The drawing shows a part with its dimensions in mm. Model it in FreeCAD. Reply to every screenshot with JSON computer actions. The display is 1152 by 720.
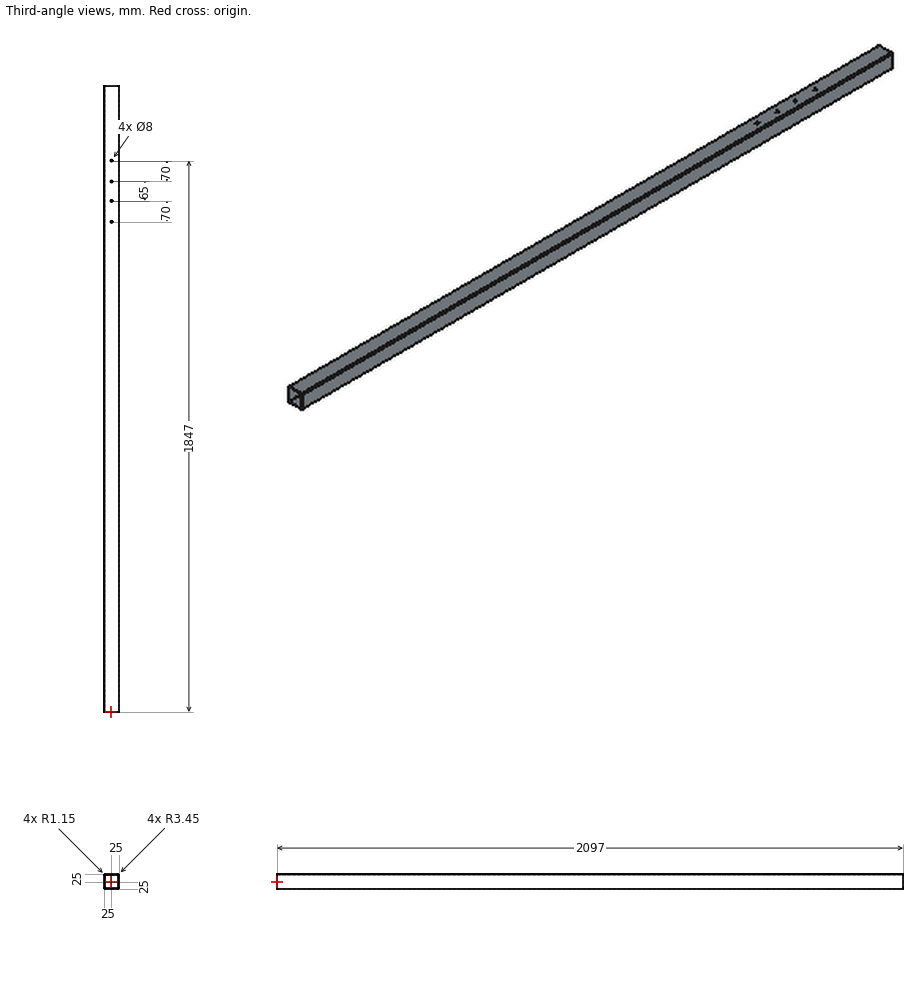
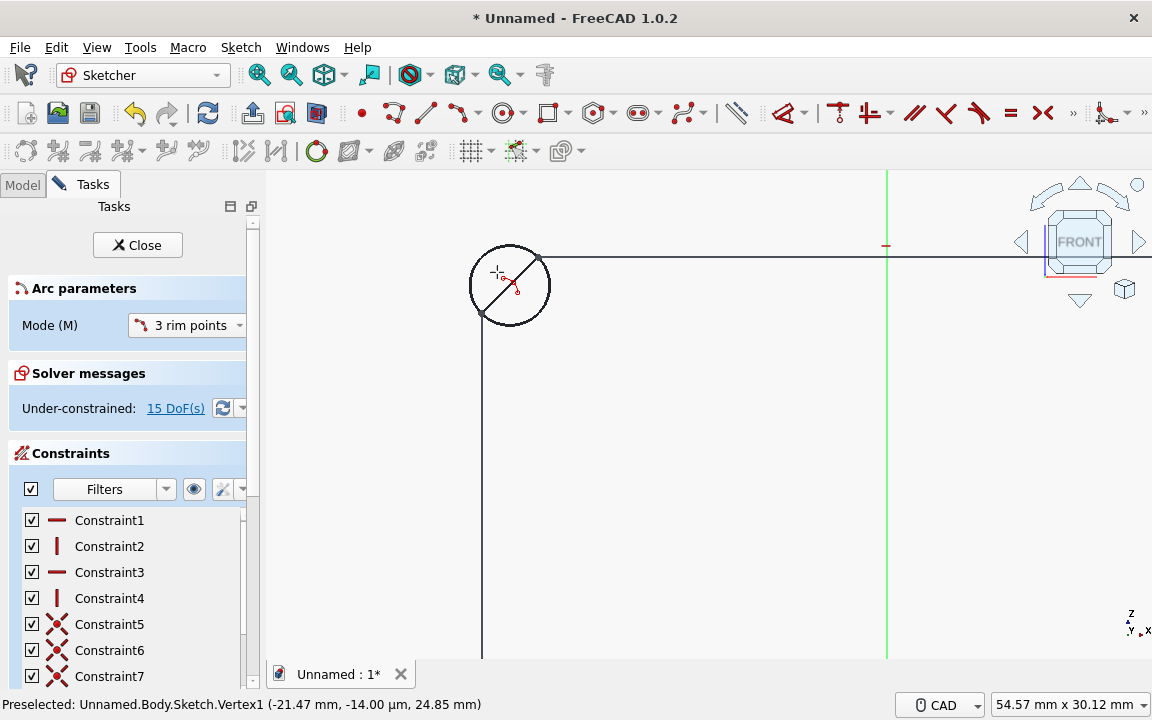
{"action": "left_click", "coordinate": [497, 271]}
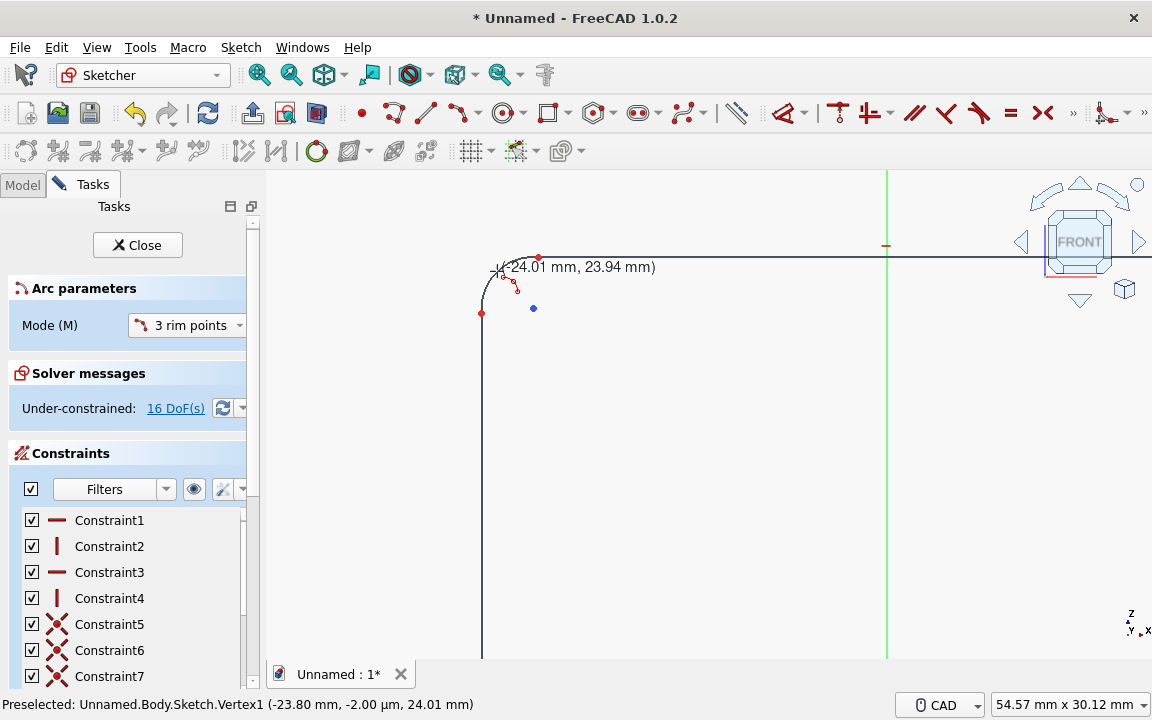
{"action": "left_click", "coordinate": [426, 114]}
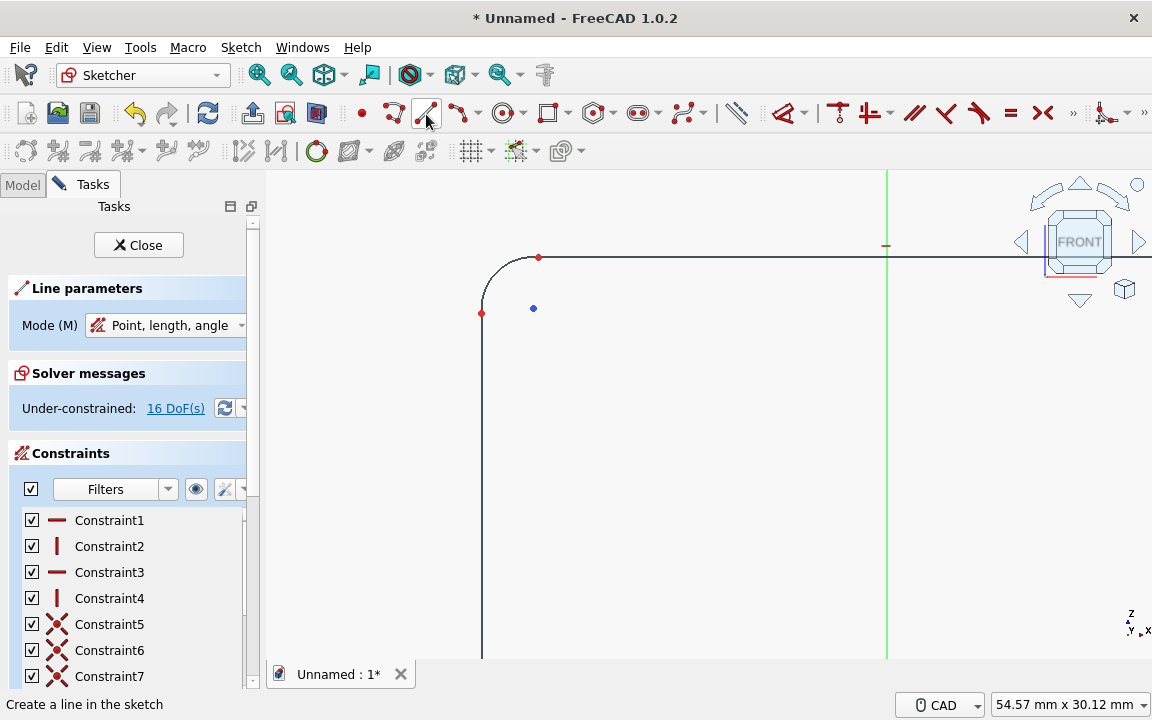
{"action": "scroll", "coordinate": [497, 271], "scroll_direction": "down", "scroll_amount": 5}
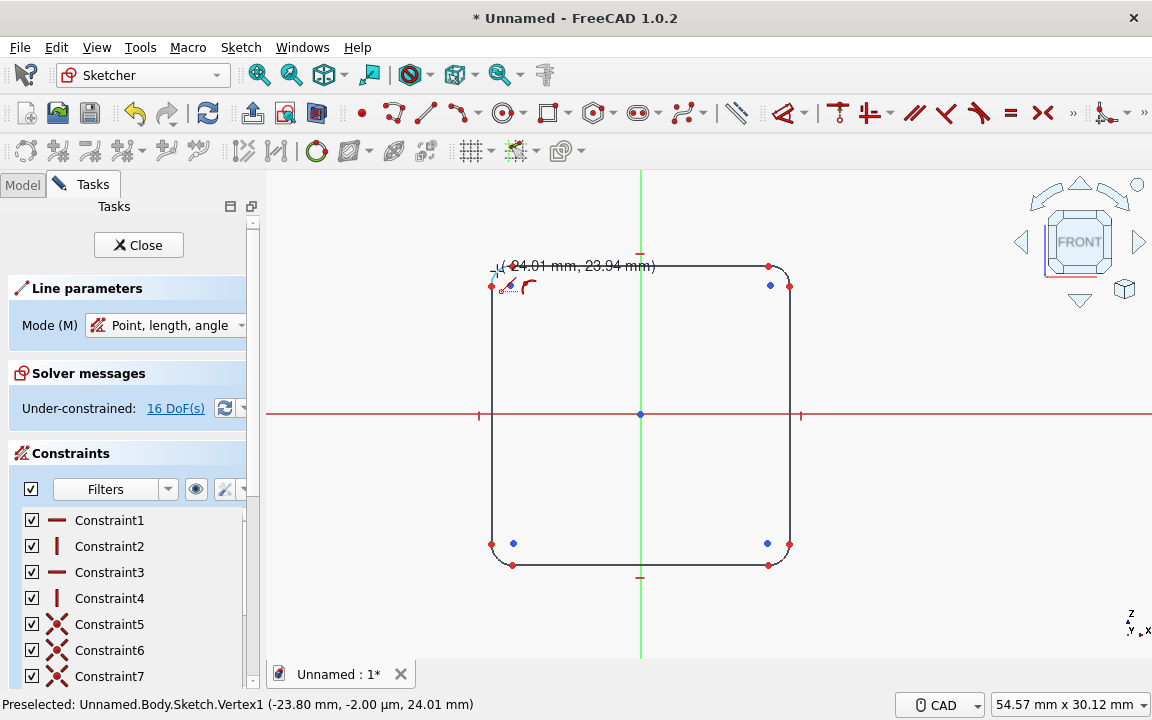
{"action": "scroll", "coordinate": [769, 279], "scroll_direction": "up", "scroll_amount": 5}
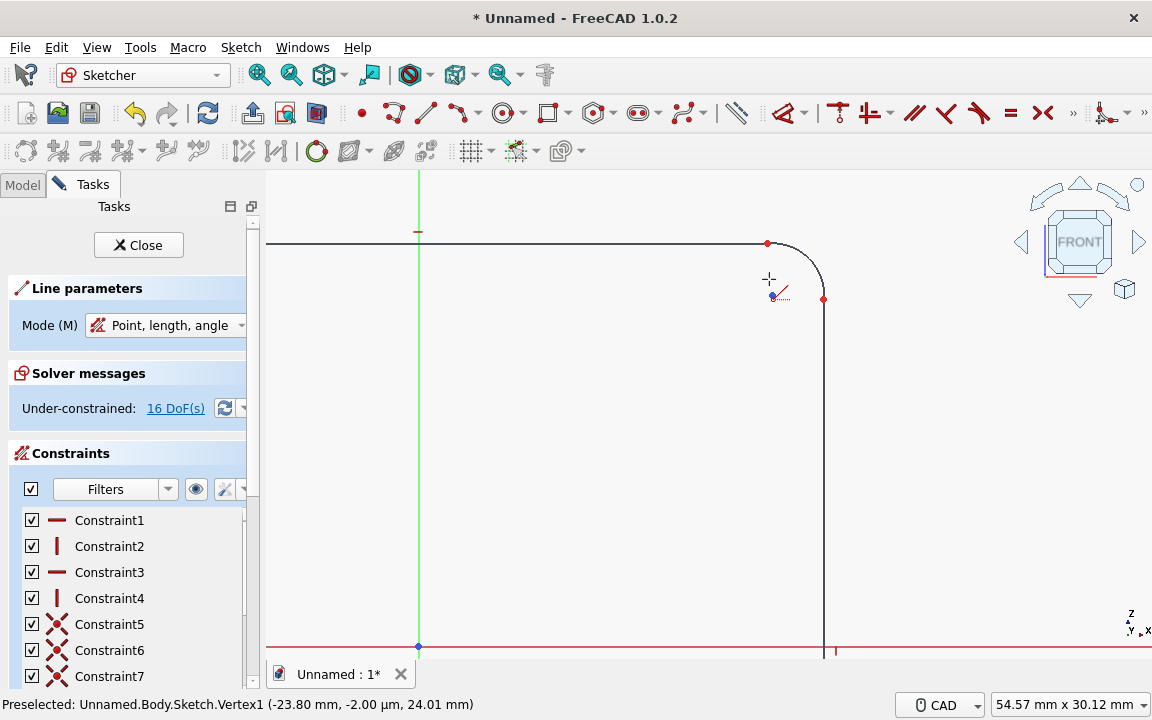
{"action": "left_click", "coordinate": [769, 278]}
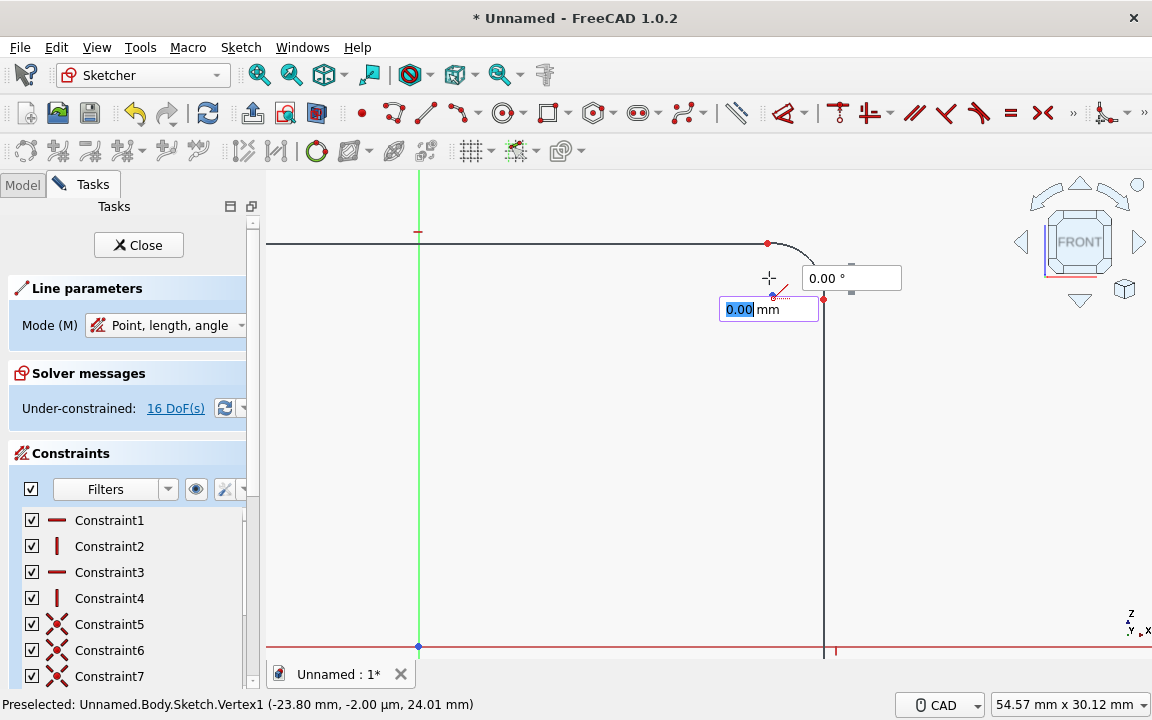
{"action": "scroll", "coordinate": [769, 279], "scroll_direction": "down", "scroll_amount": 5}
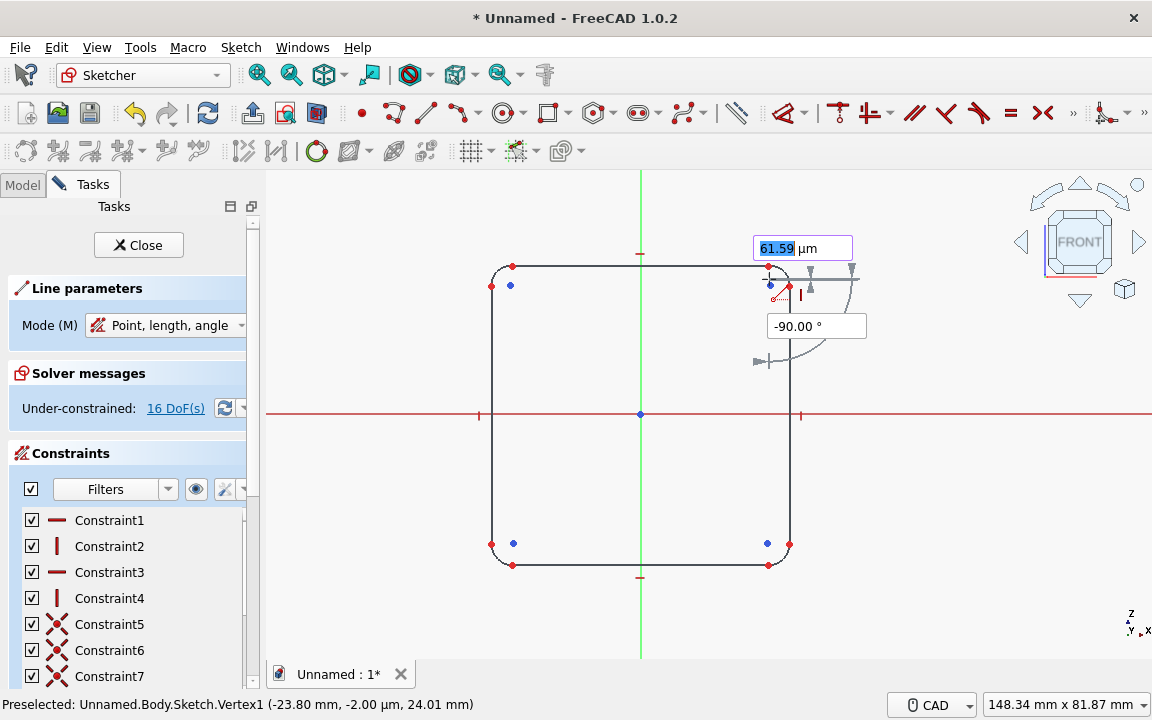
{"action": "scroll", "coordinate": [512, 279], "scroll_direction": "up", "scroll_amount": 5}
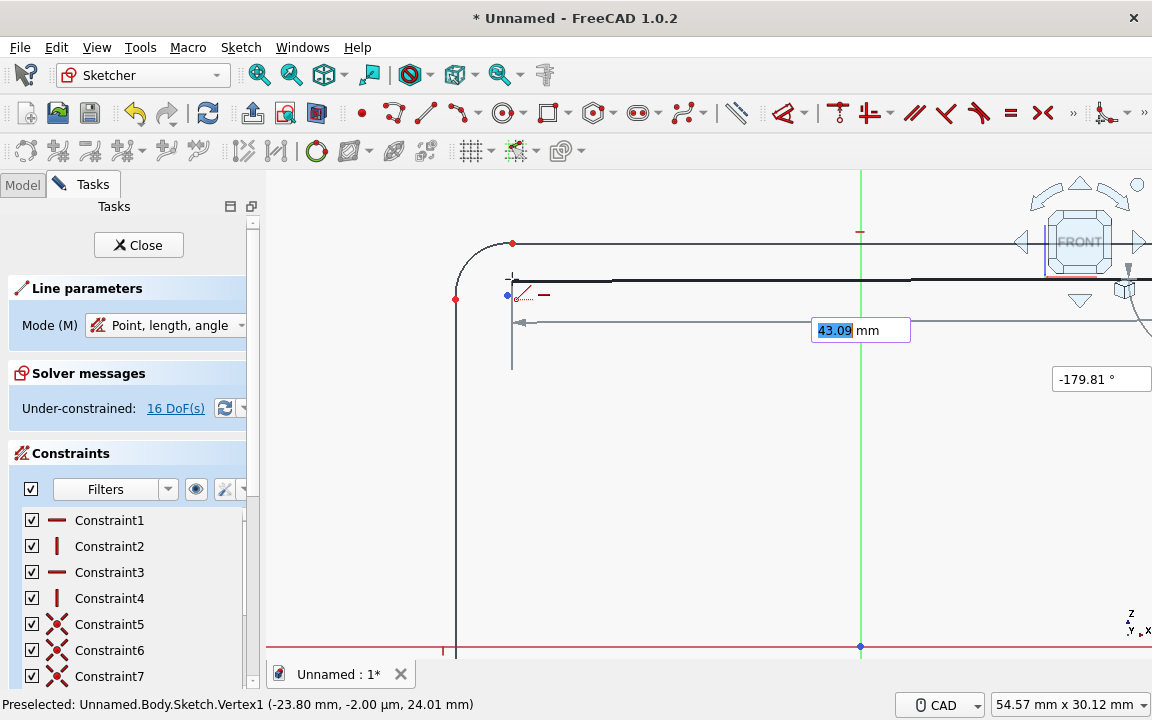
{"action": "left_click", "coordinate": [511, 278]}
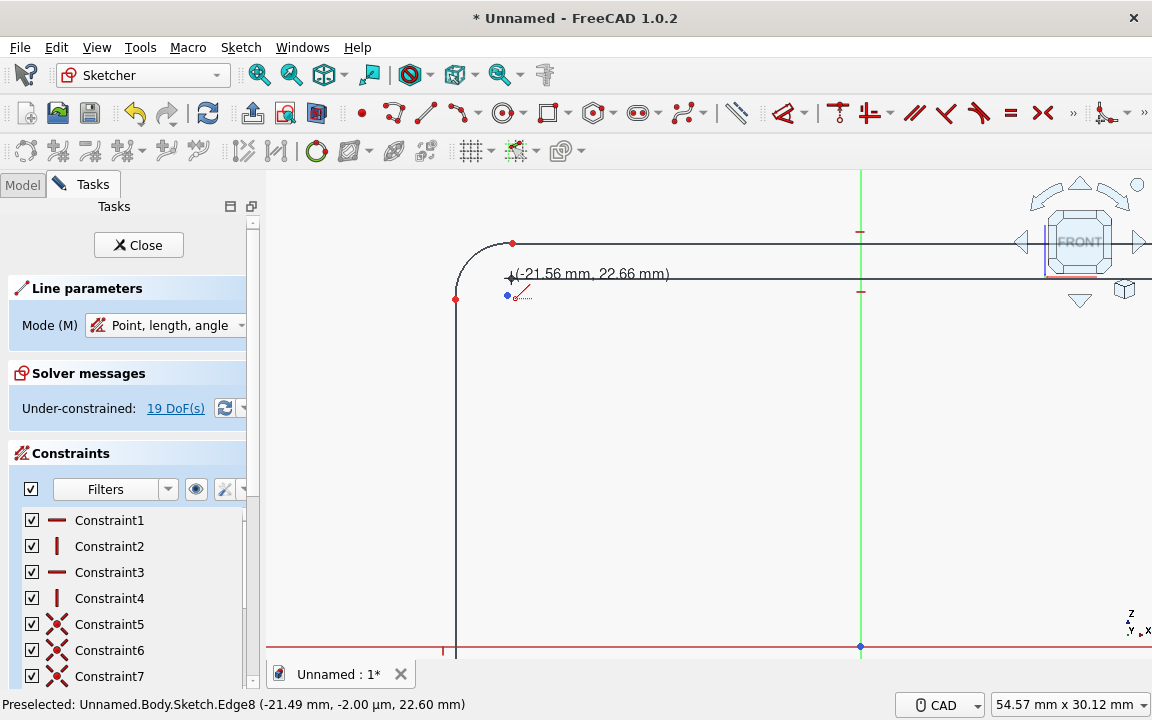
{"action": "left_click", "coordinate": [492, 297]}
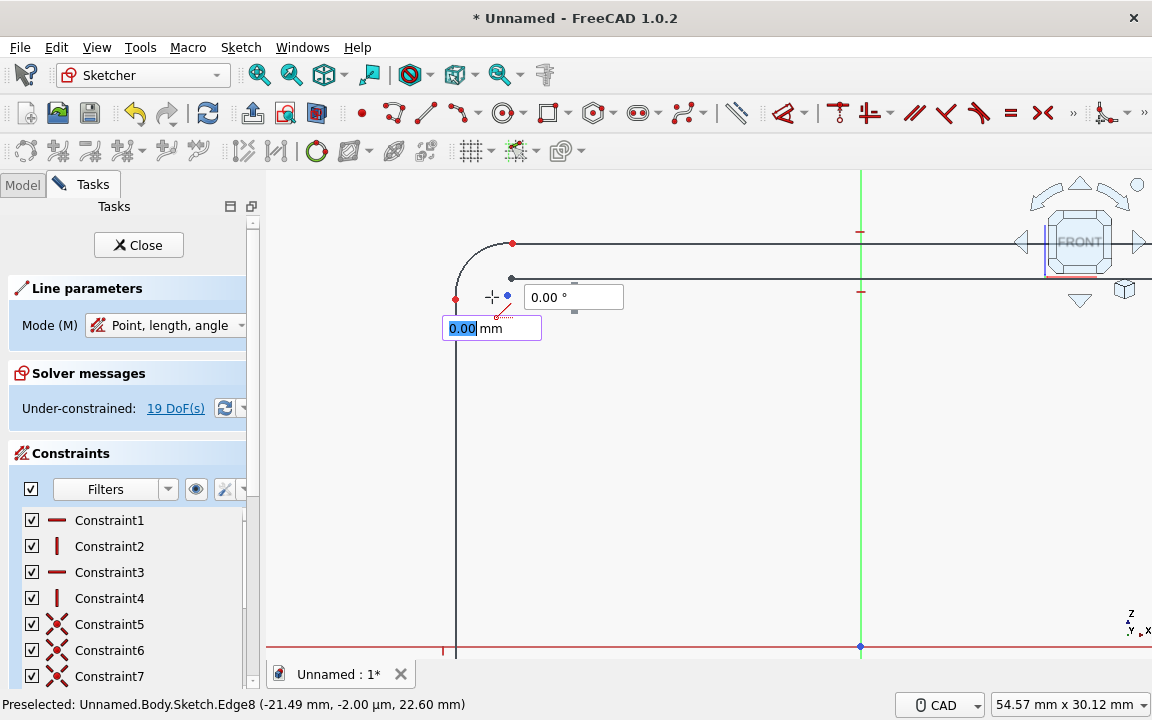
{"action": "scroll", "coordinate": [512, 279], "scroll_direction": "down", "scroll_amount": 5}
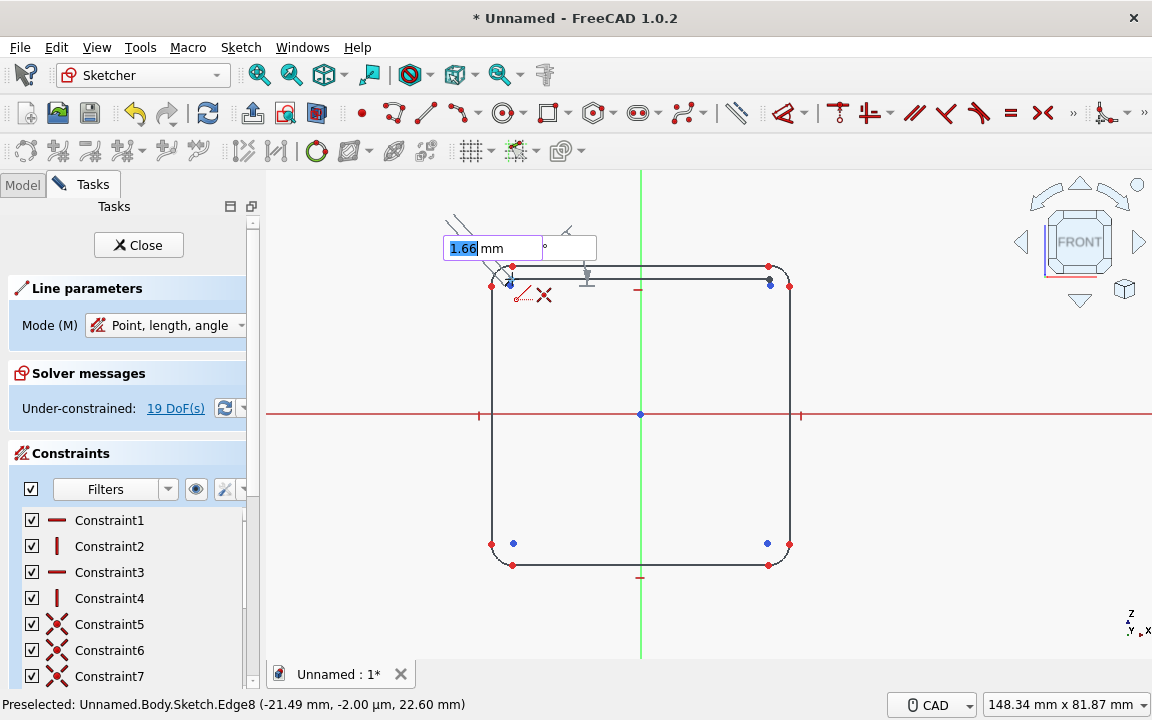
{"action": "scroll", "coordinate": [505, 543], "scroll_direction": "up", "scroll_amount": 5}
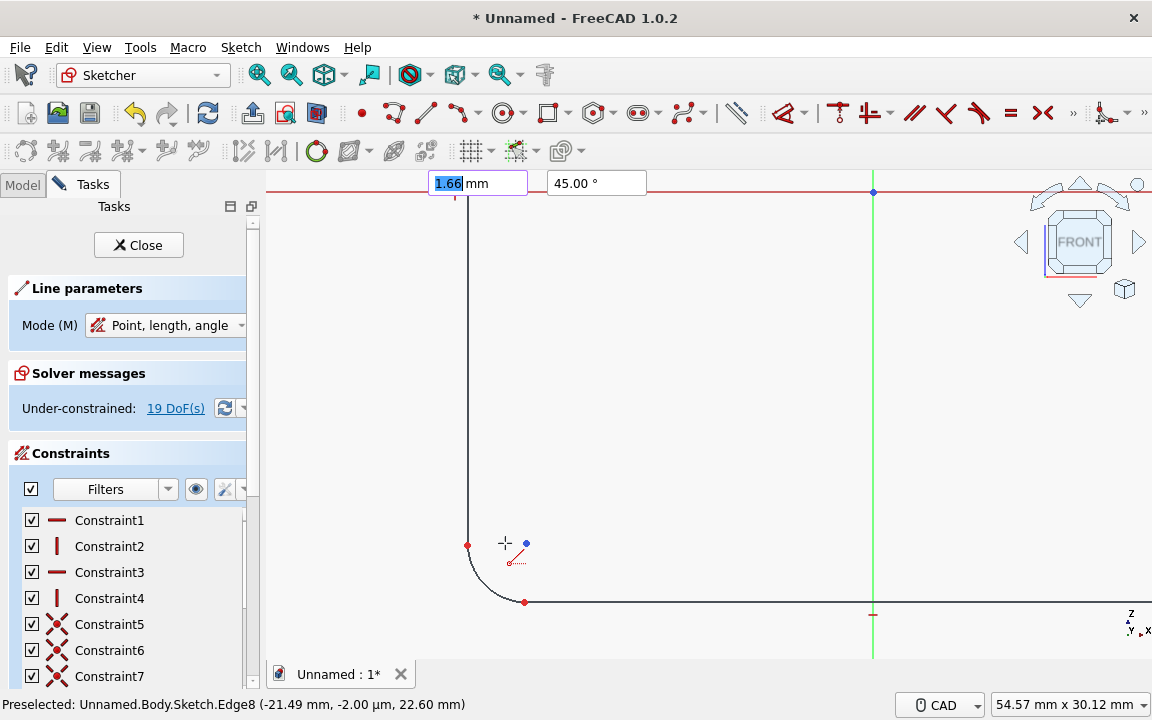
{"action": "left_click", "coordinate": [504, 542]}